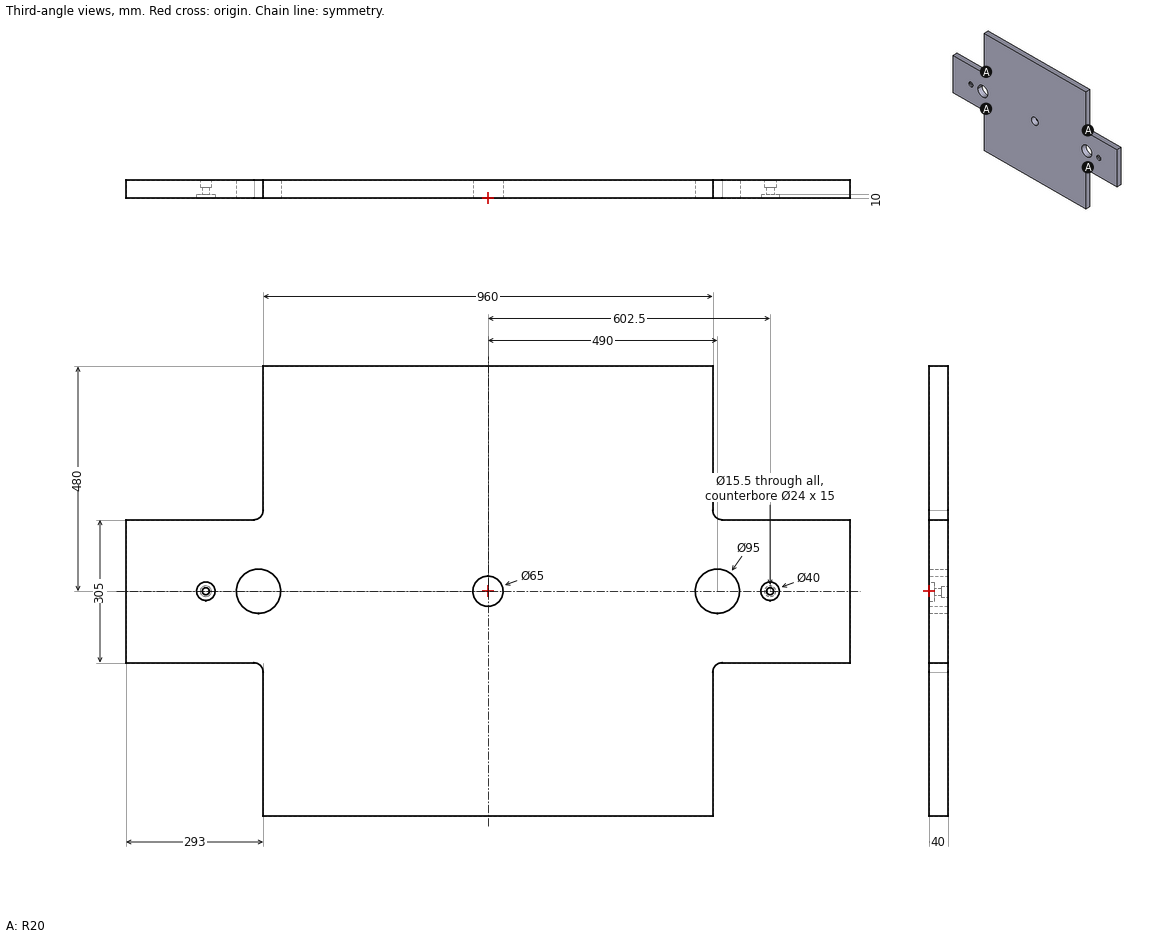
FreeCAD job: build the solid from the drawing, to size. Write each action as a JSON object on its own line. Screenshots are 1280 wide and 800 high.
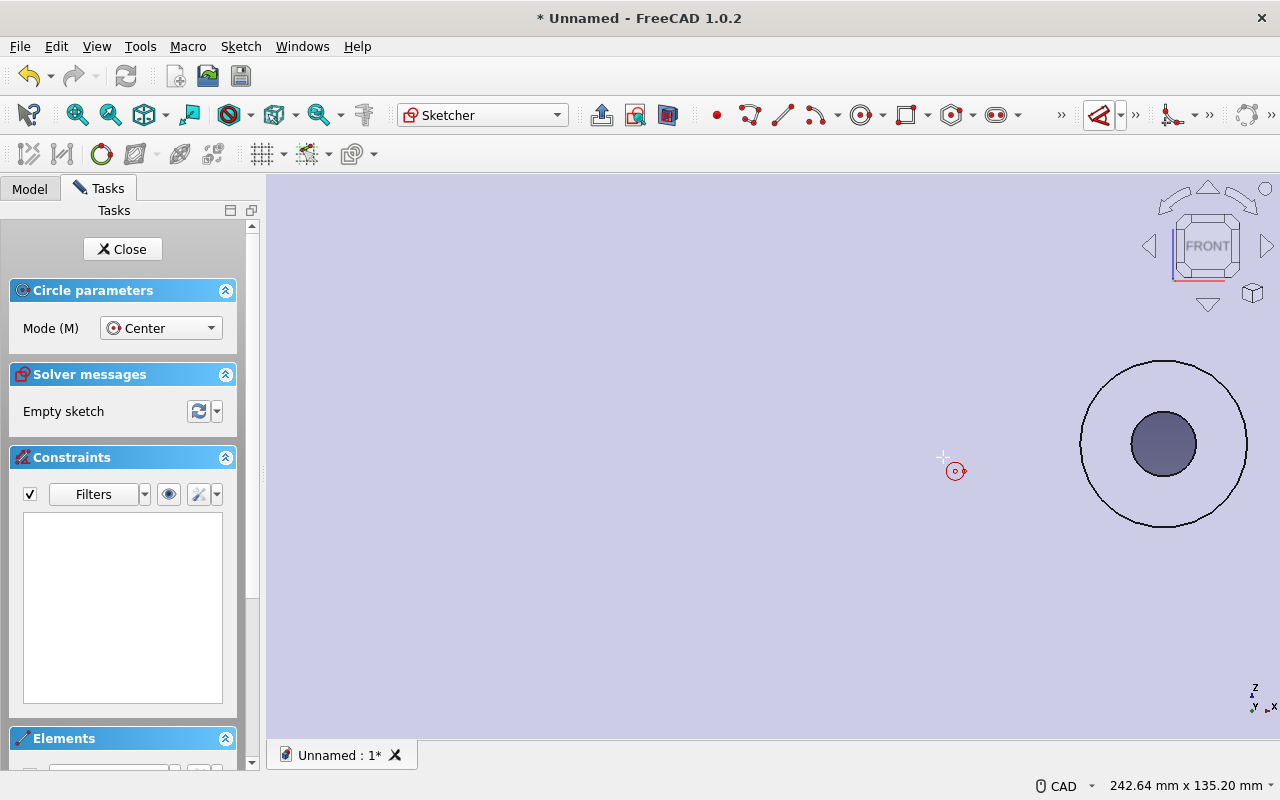
{"action": "left_click", "coordinate": [694, 444]}
{"action": "mouse_move", "coordinate": [834, 304]}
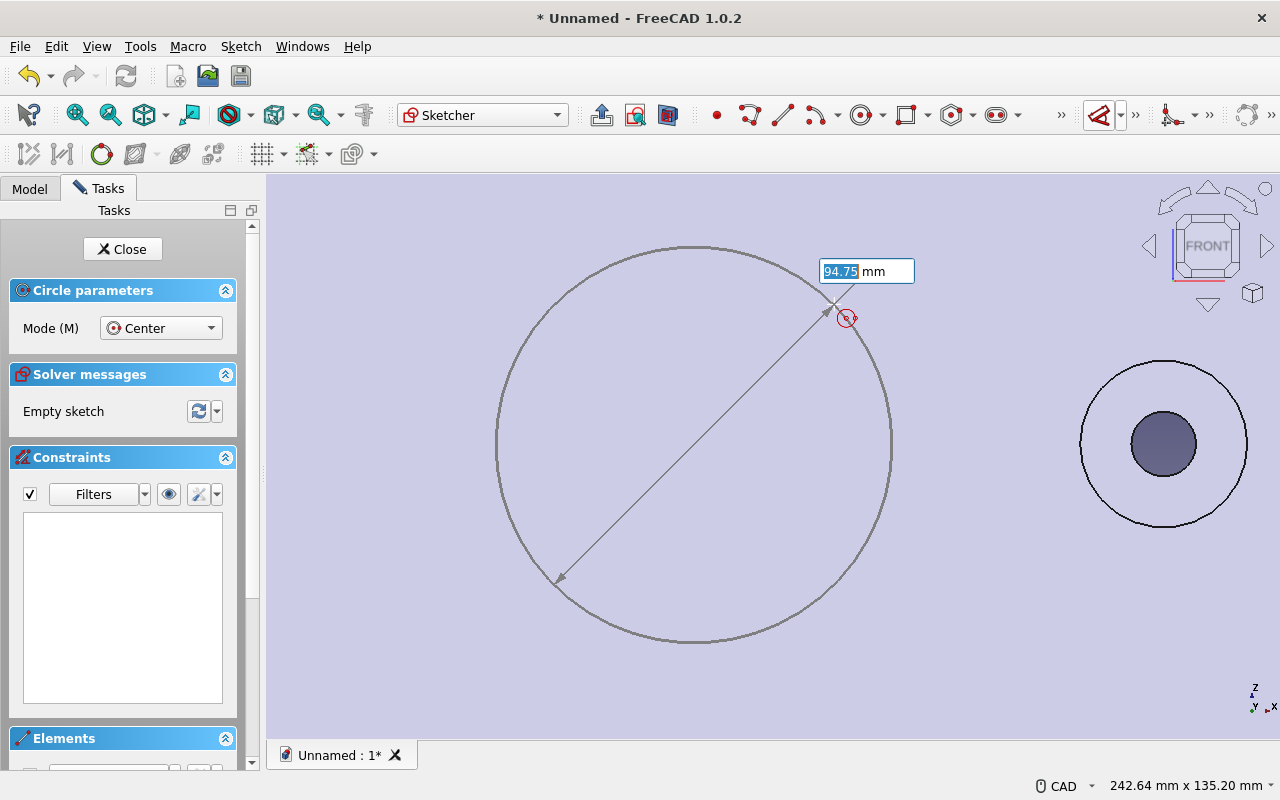
{"action": "type", "text": "95"}
{"action": "key", "text": "Return"}
{"action": "key", "text": "Escape"}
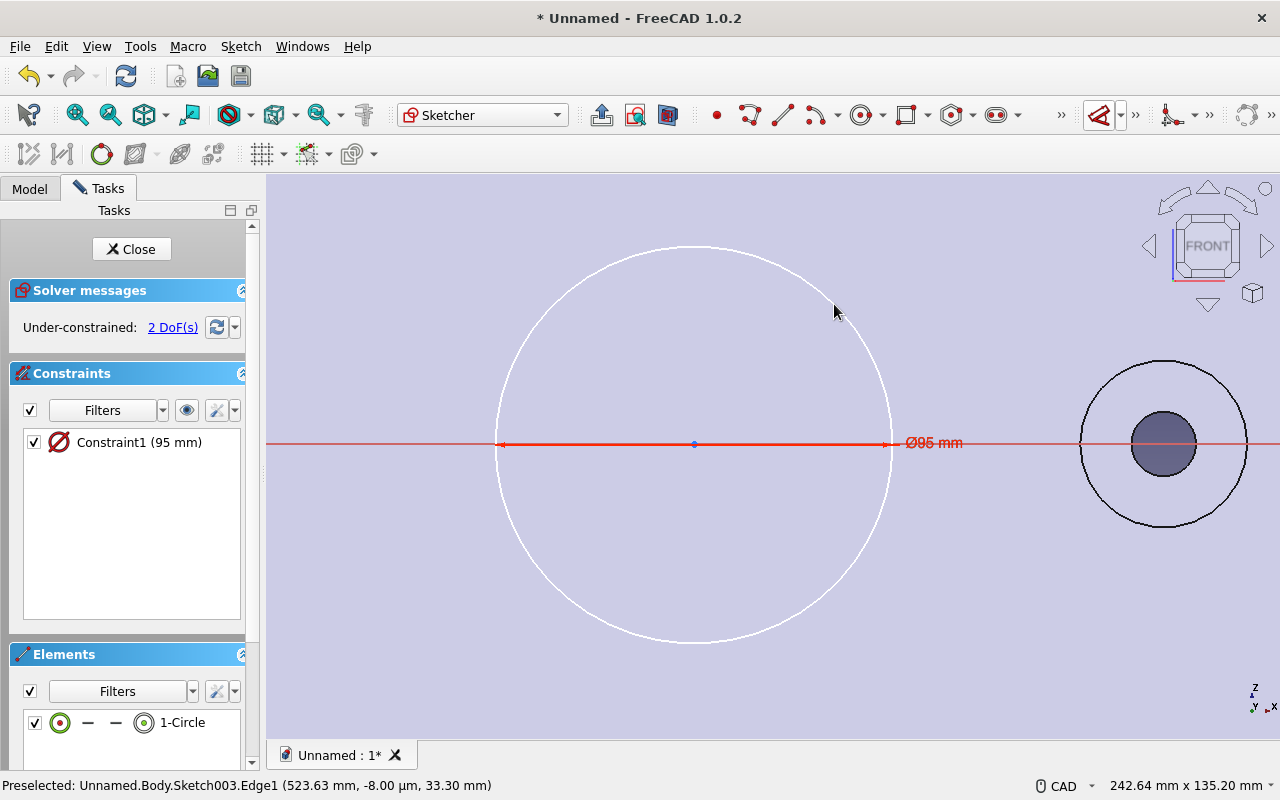
{"action": "left_click", "coordinate": [694, 445]}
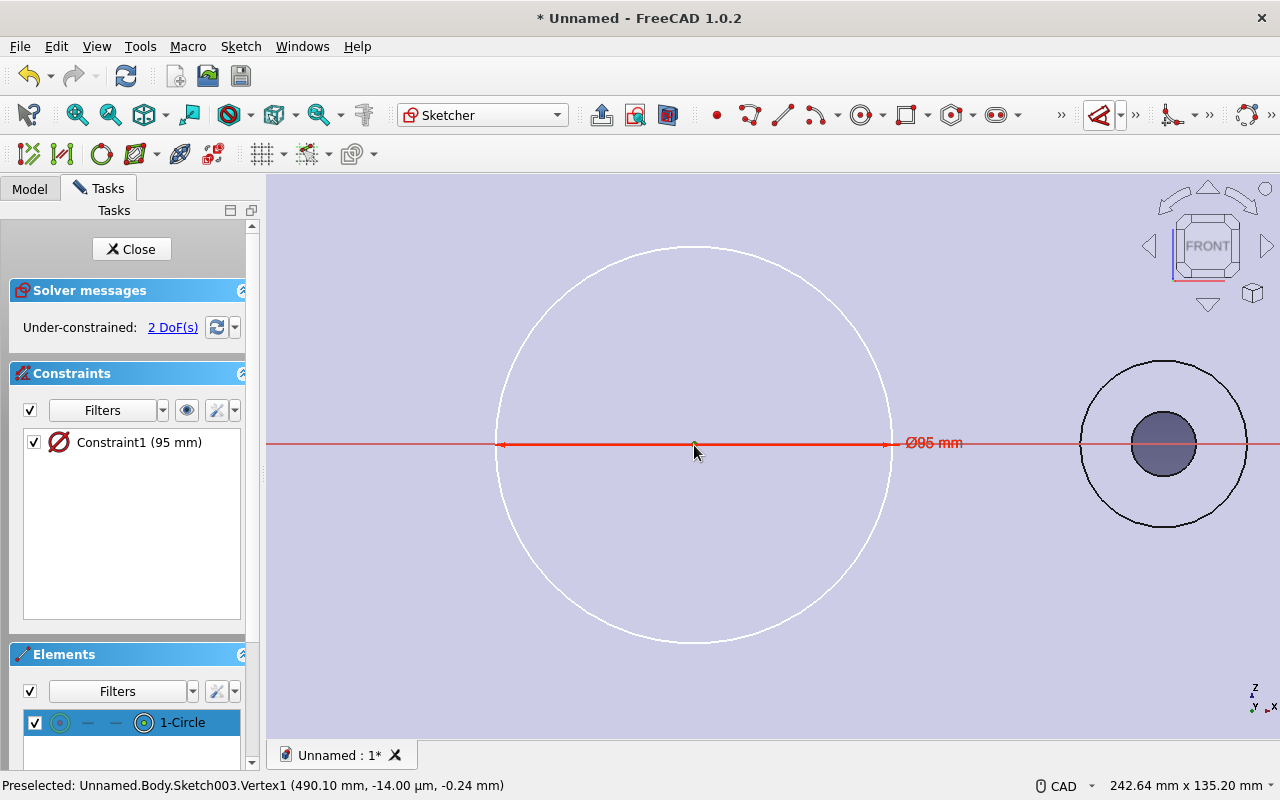
{"action": "left_click", "coordinate": [353, 444]}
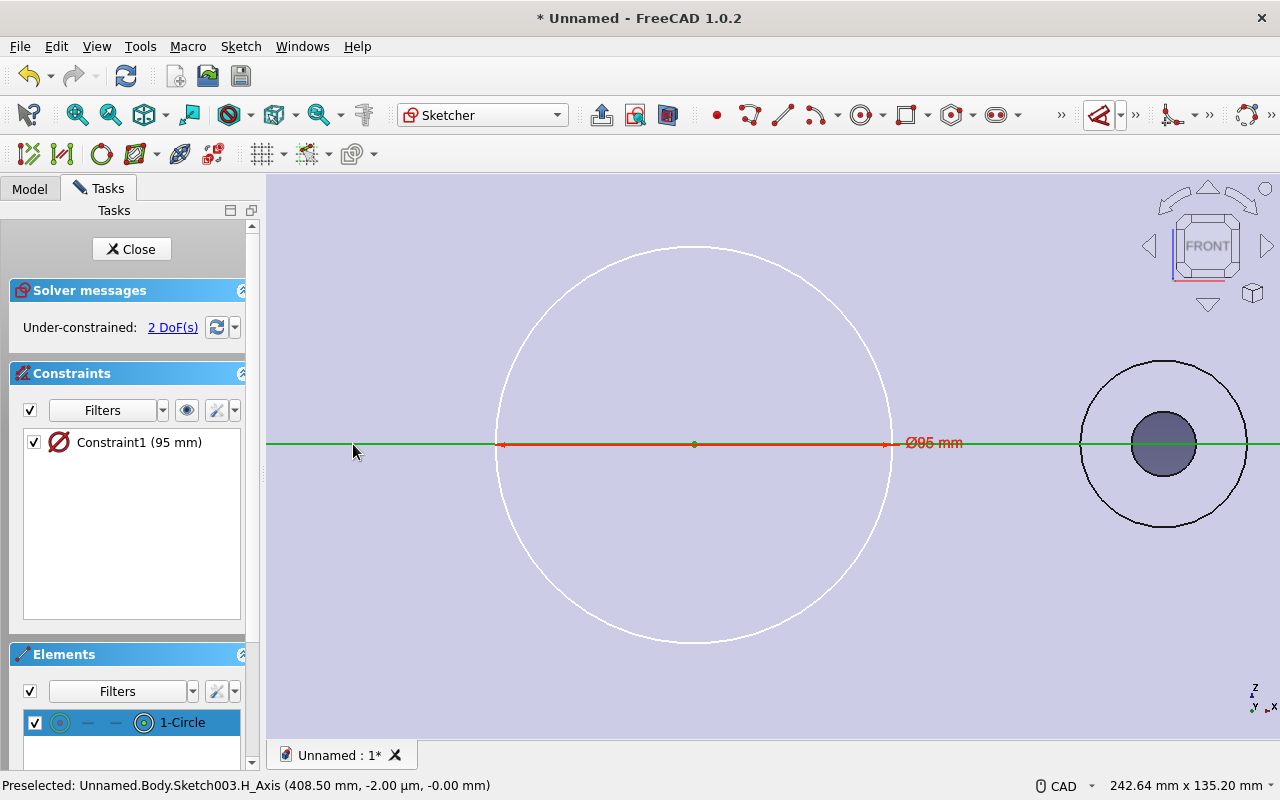
{"action": "key", "text": "c"}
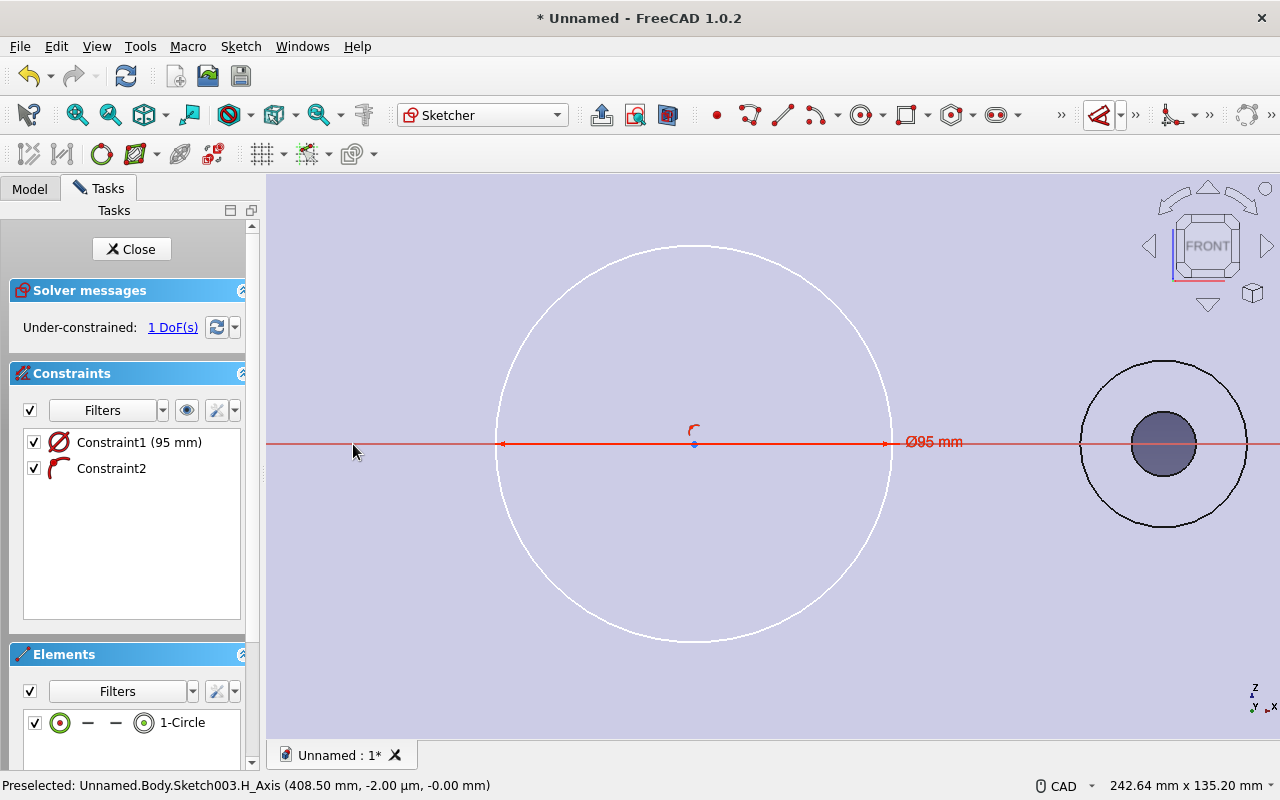
{"action": "left_click", "coordinate": [694, 444]}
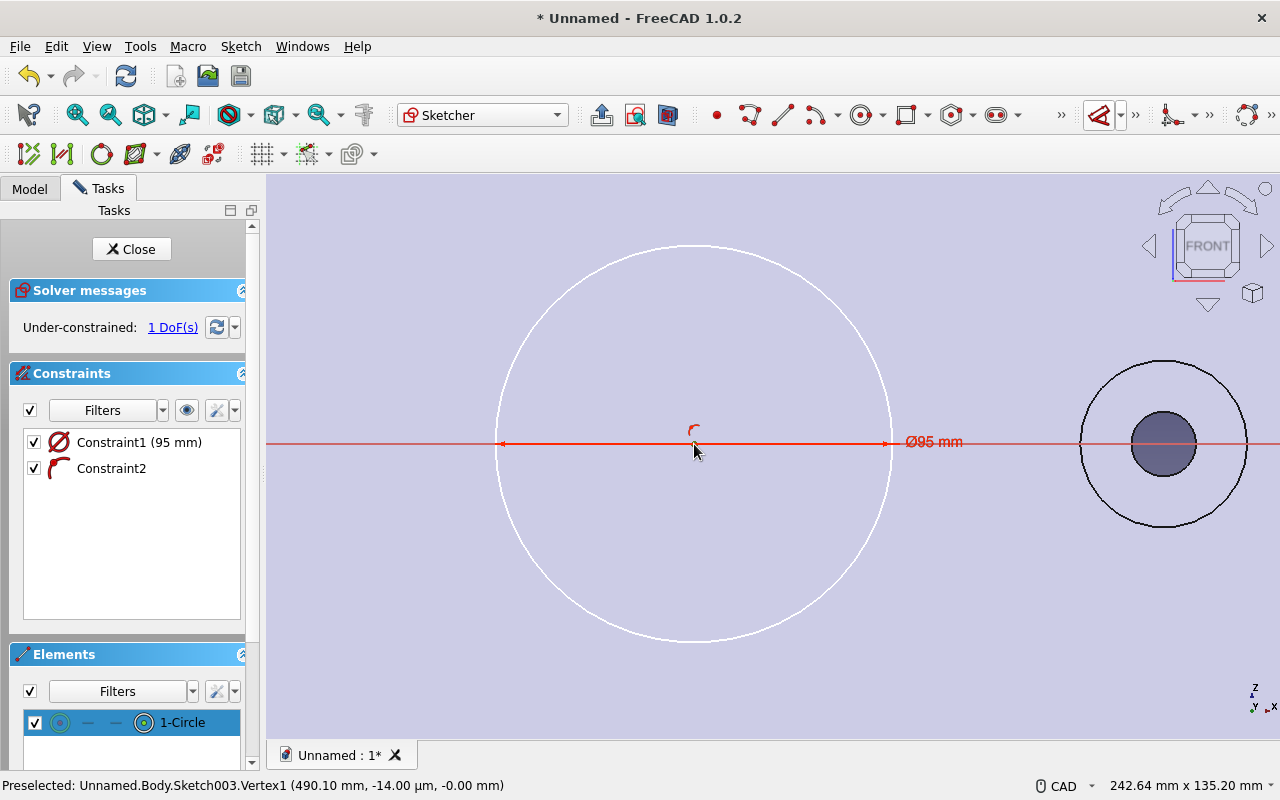
{"action": "key", "text": "l"}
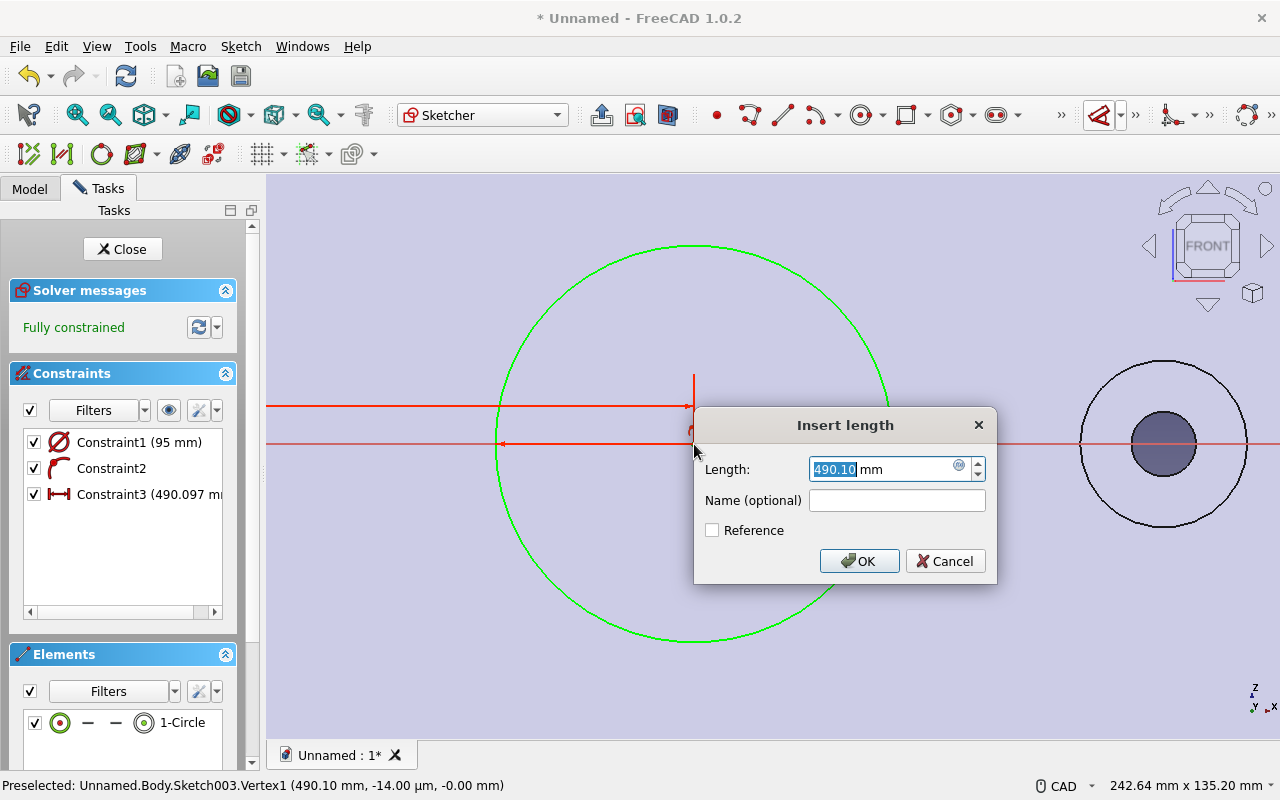
{"action": "type", "text": "490"}
{"action": "key", "text": "Return"}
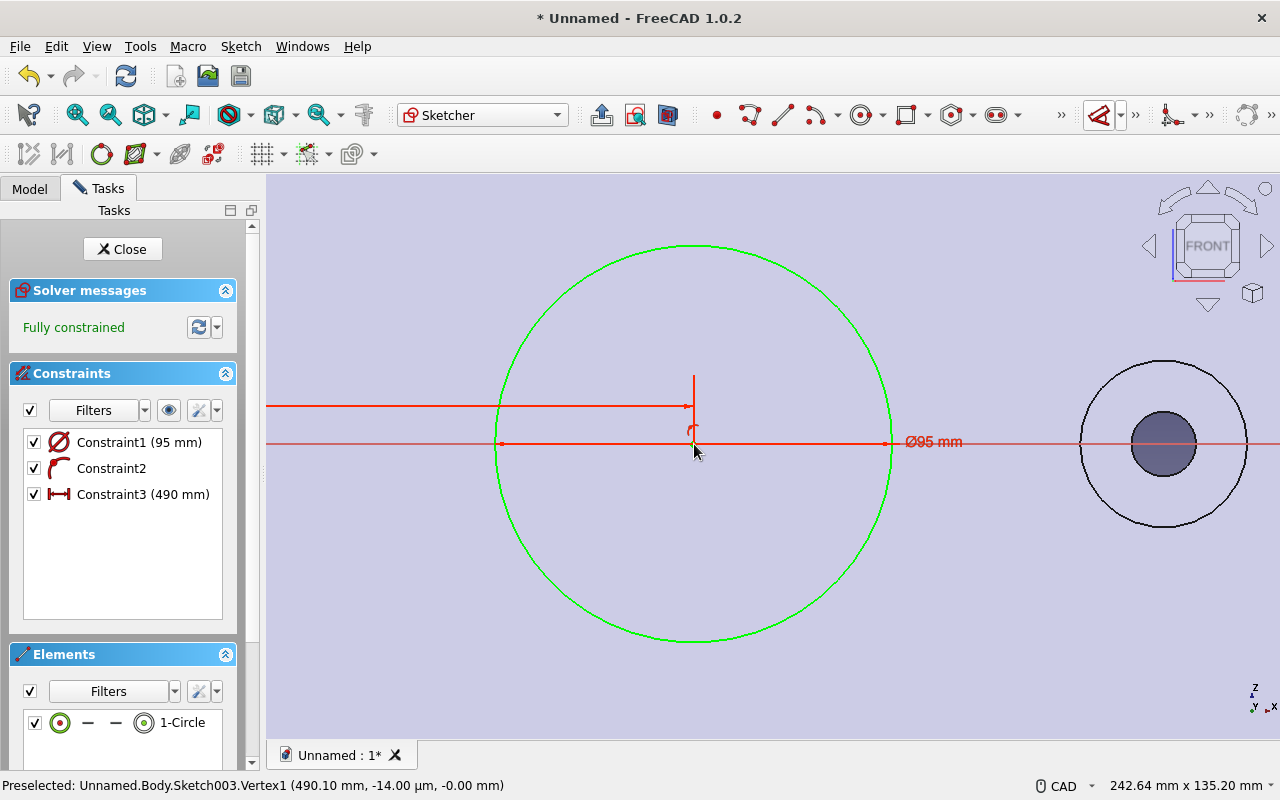
{"action": "left_click", "coordinate": [123, 249]}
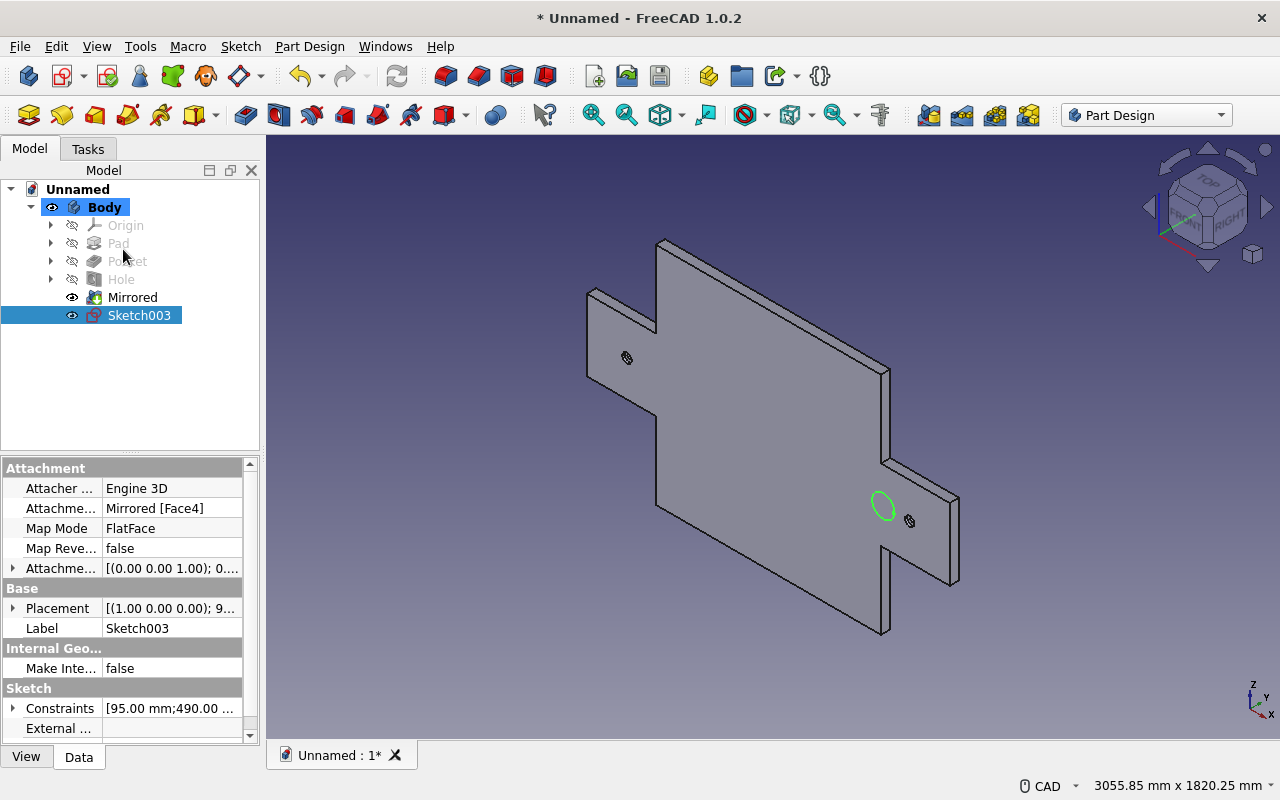
{"action": "left_click", "coordinate": [246, 116]}